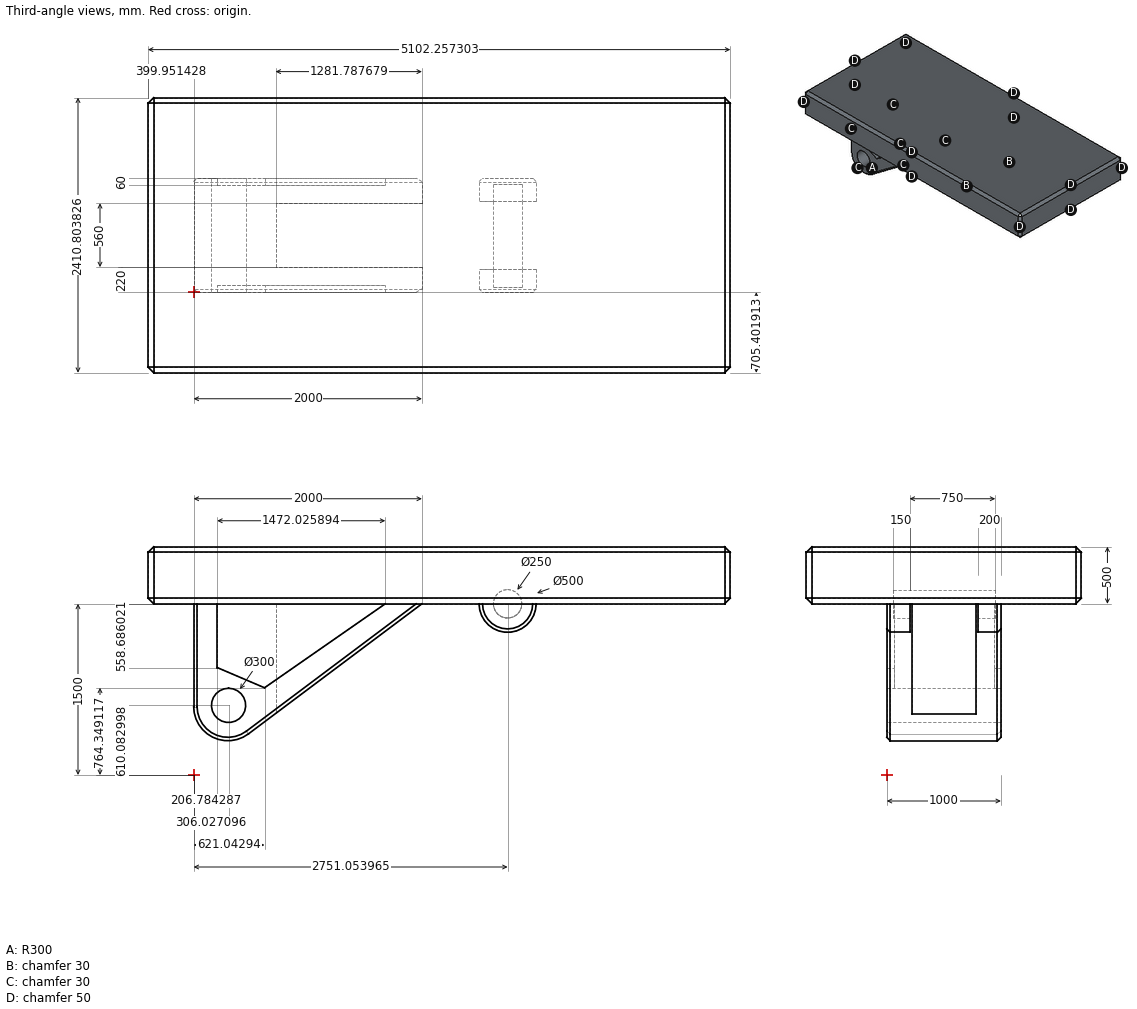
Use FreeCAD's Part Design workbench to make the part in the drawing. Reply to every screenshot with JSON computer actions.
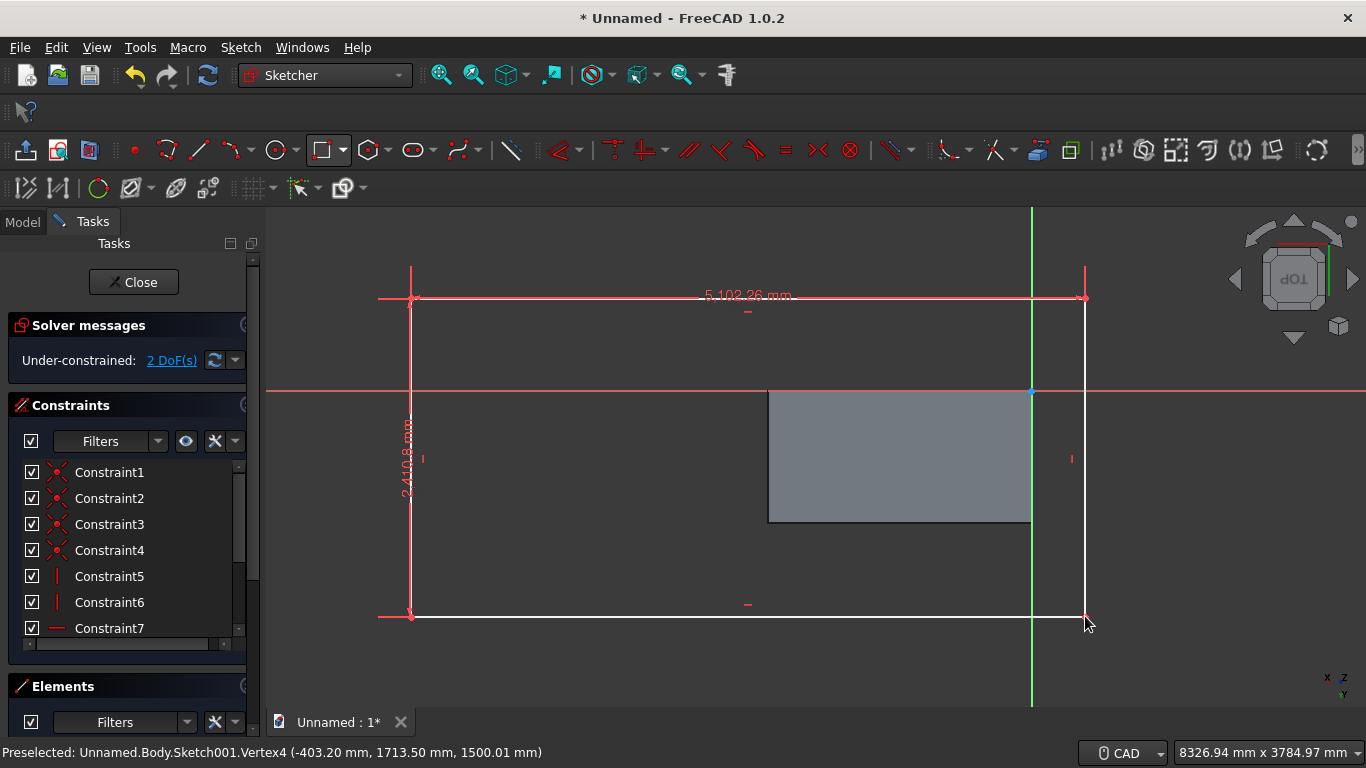
{"action": "key", "text": "d"}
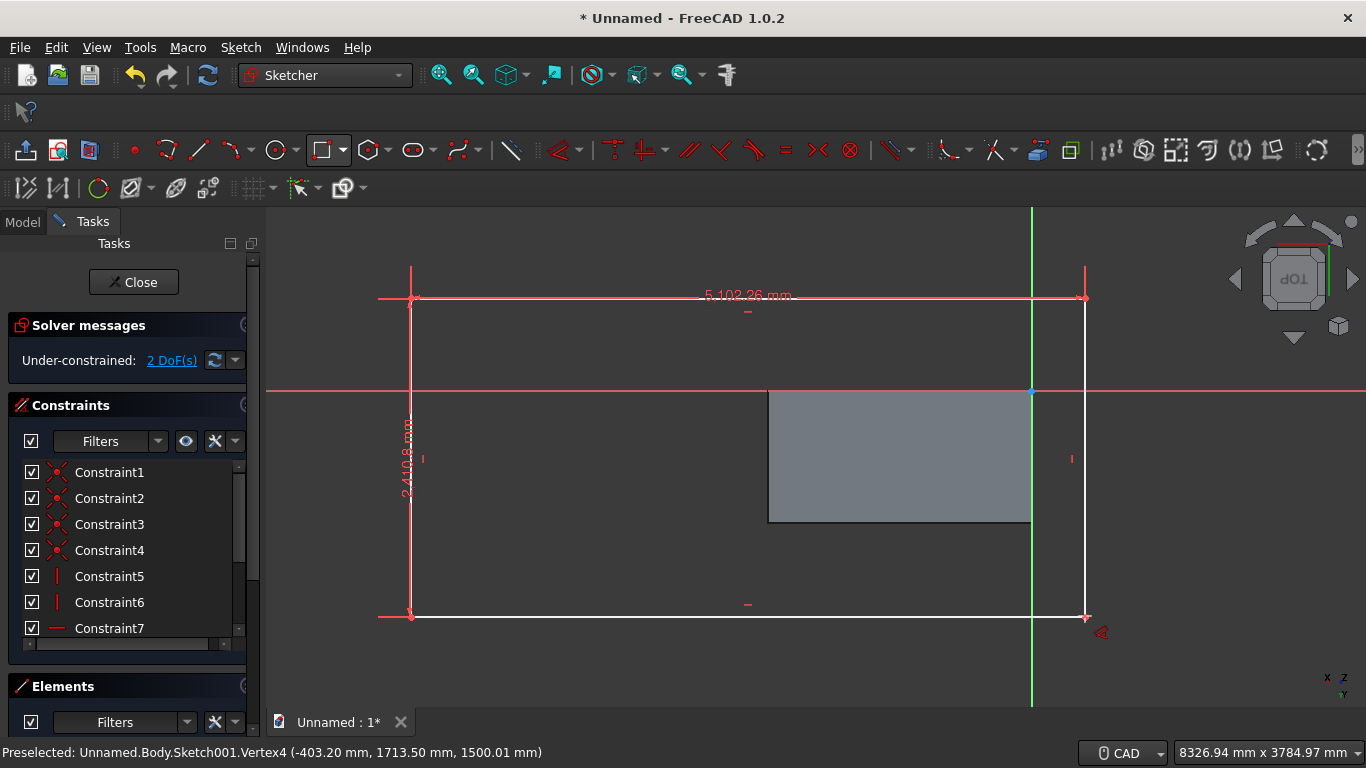
{"action": "left_click", "coordinate": [411, 299]}
{"action": "left_click", "coordinate": [377, 345]}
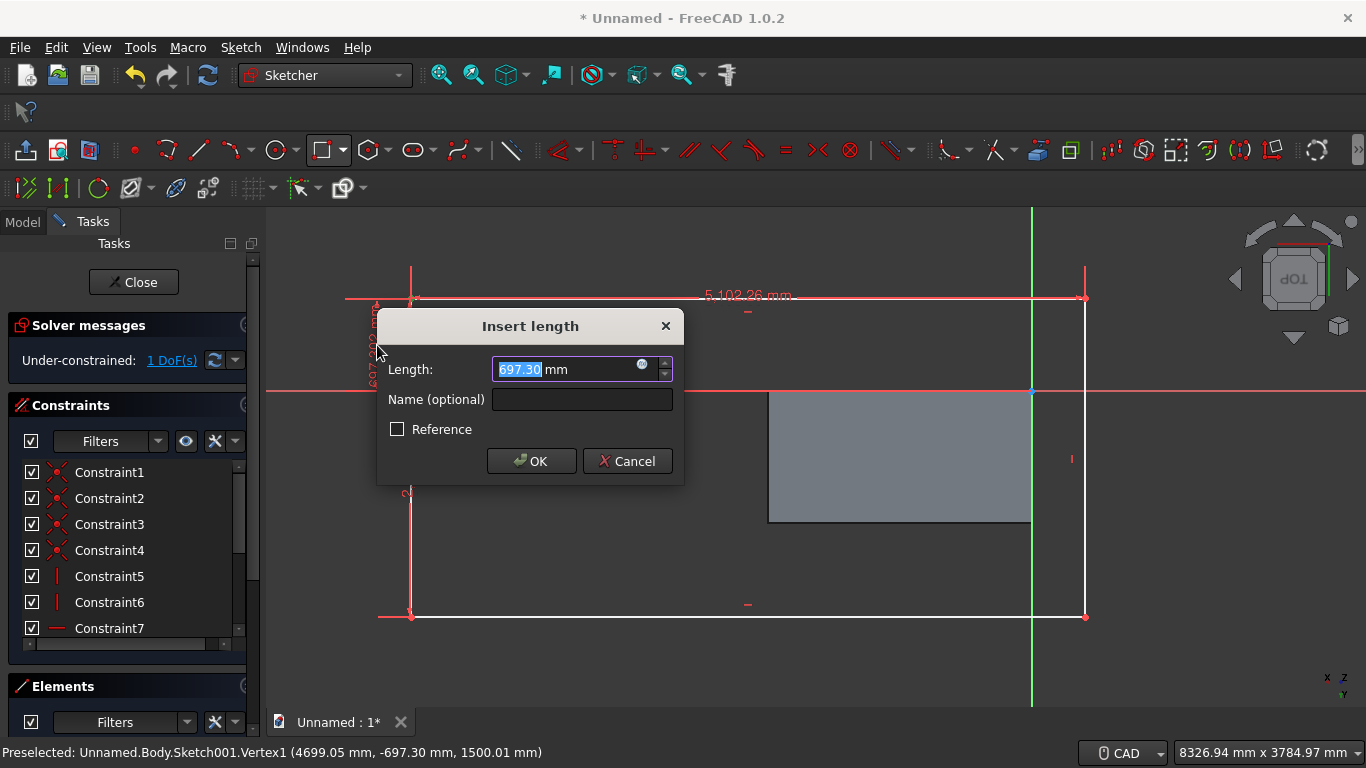
{"action": "type", "text": "705.401913"}
{"action": "key", "text": "Return"}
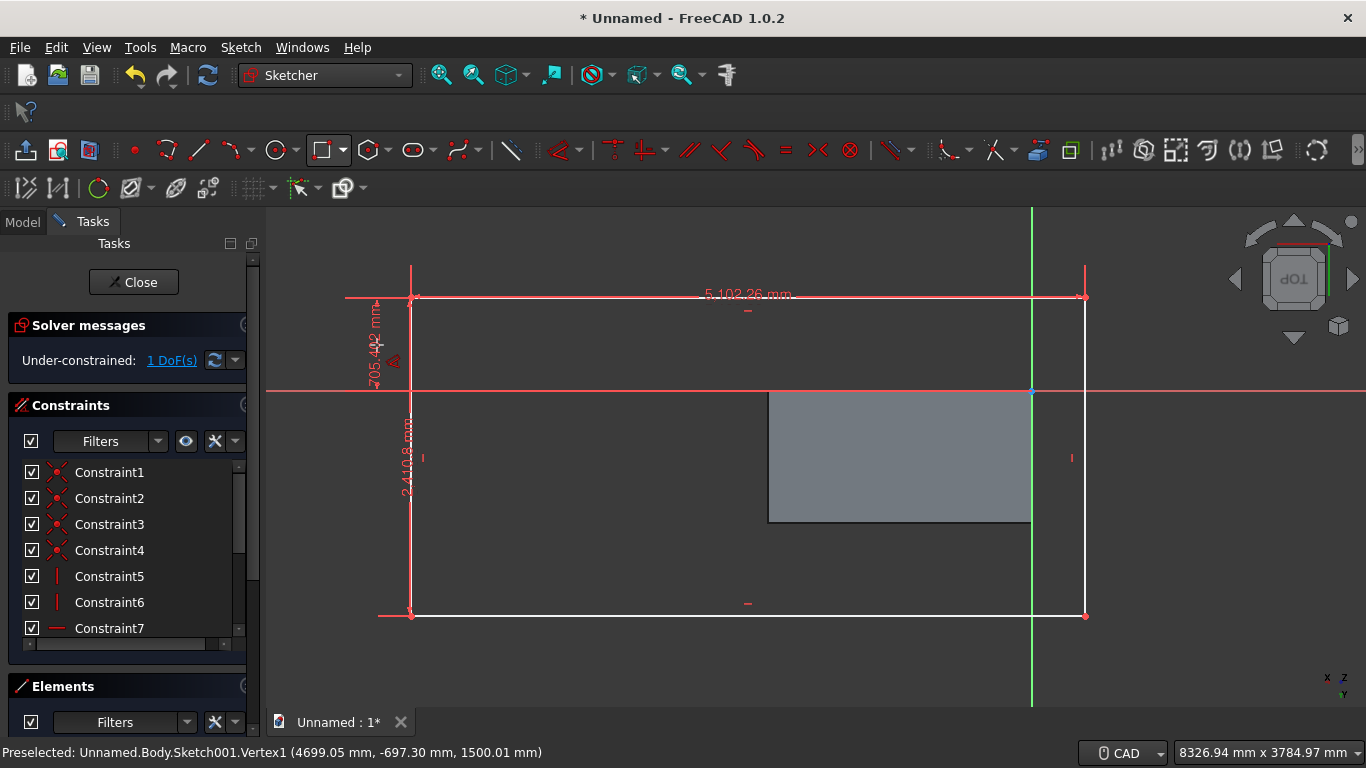
{"action": "left_click", "coordinate": [1085, 616]}
{"action": "left_click", "coordinate": [1058, 650]}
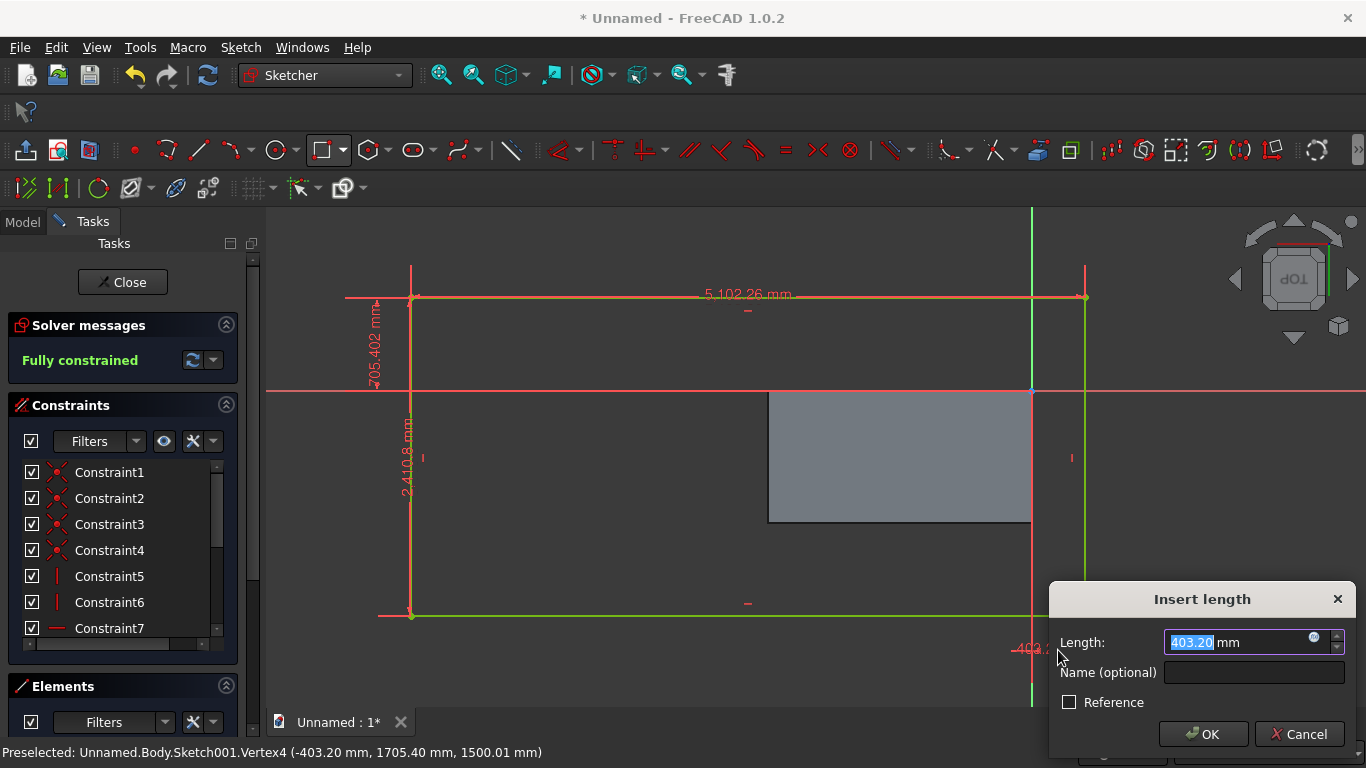
{"action": "type", "text": "399.951428"}
{"action": "key", "text": "Return"}
{"action": "key", "text": "Escape"}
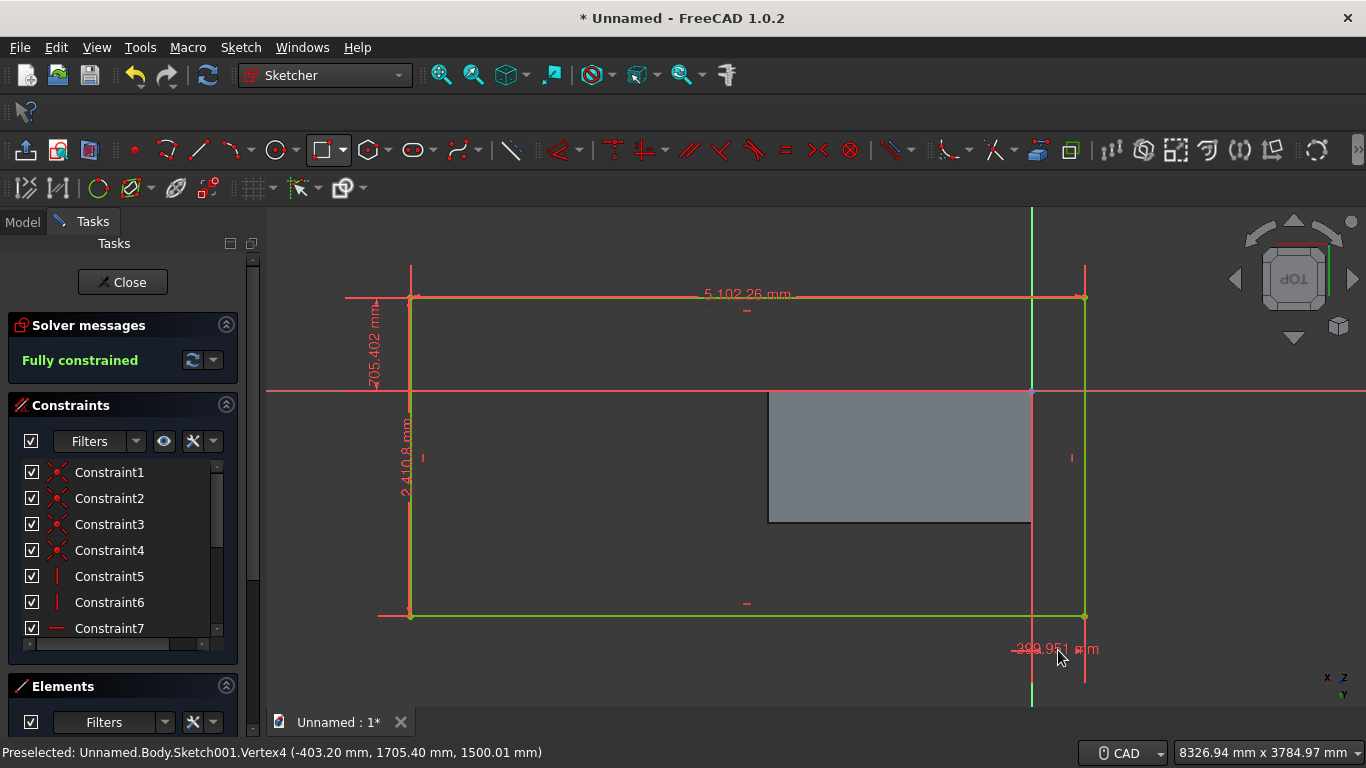
{"action": "left_click", "coordinate": [123, 282]}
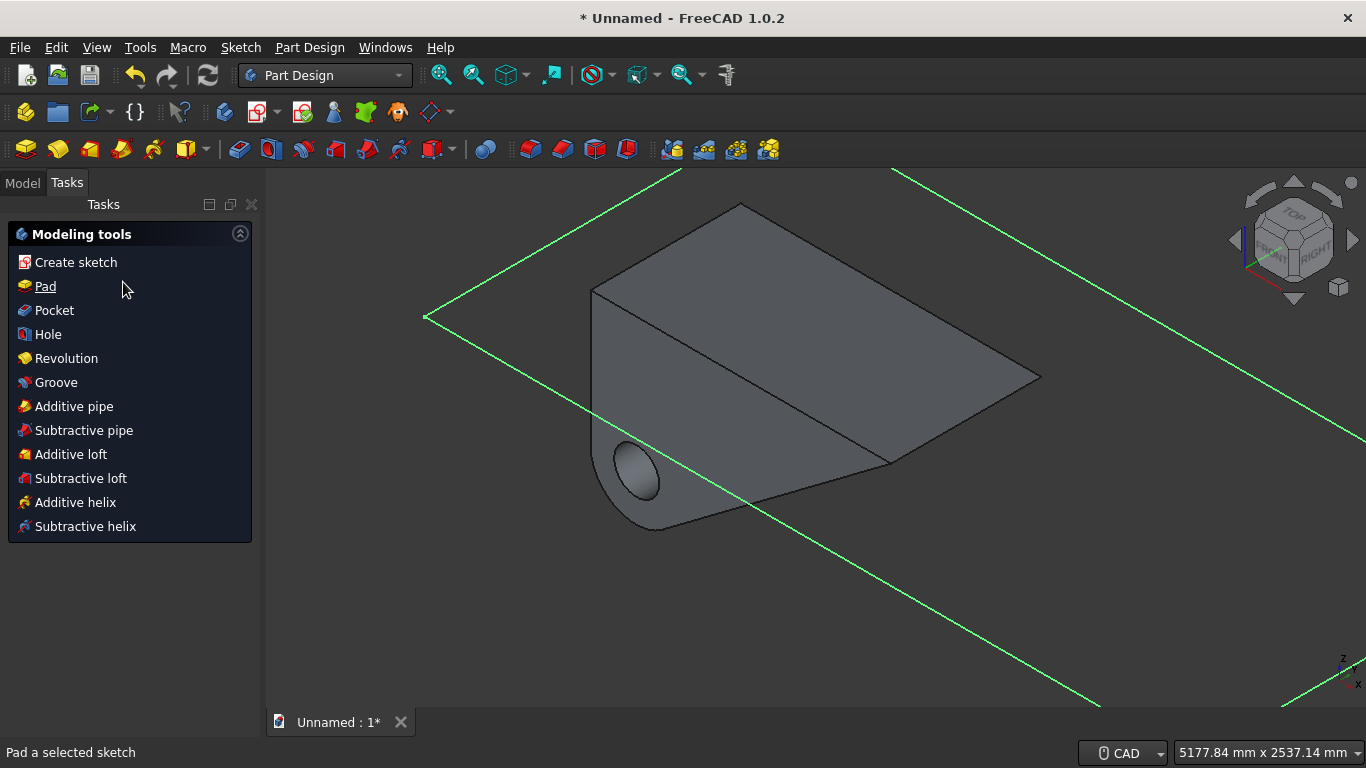
{"action": "left_click", "coordinate": [26, 150]}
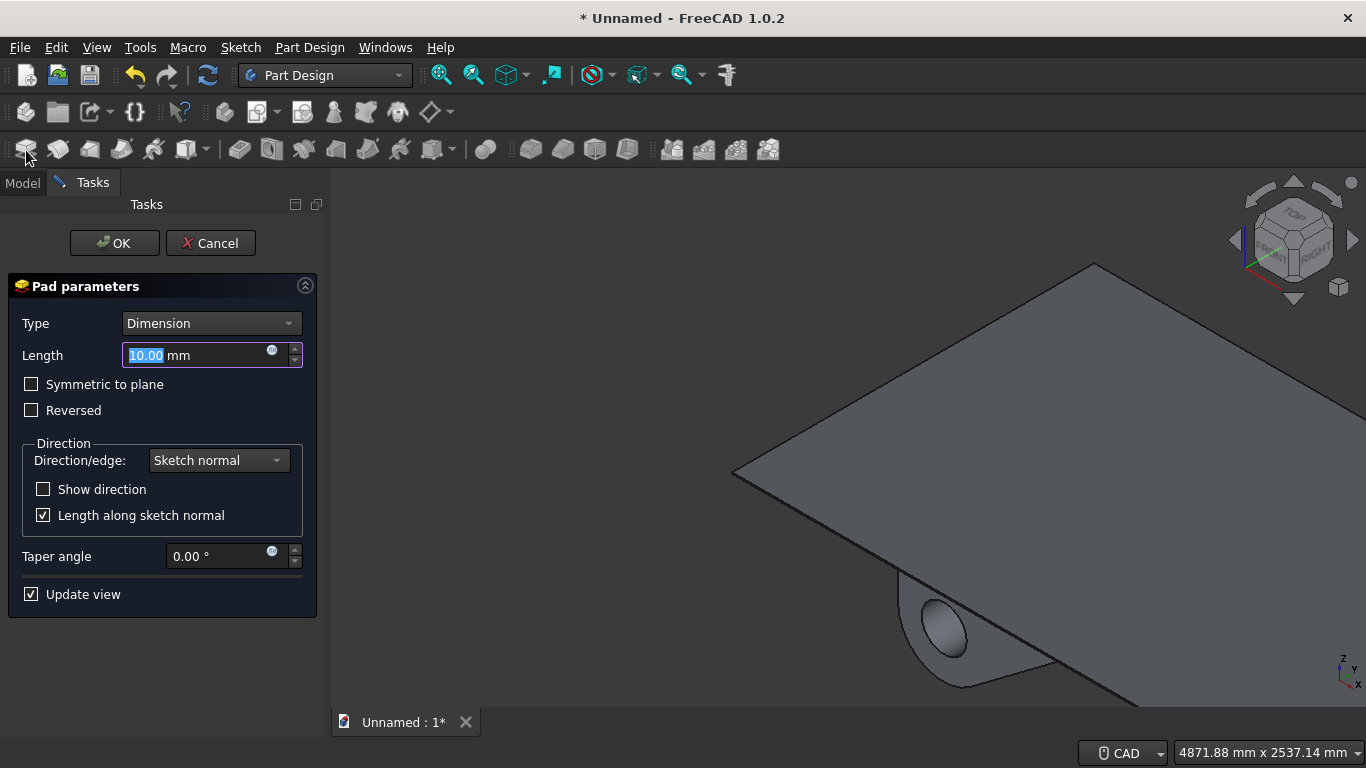
{"action": "type", "text": "500"}
{"action": "key", "text": "Tab"}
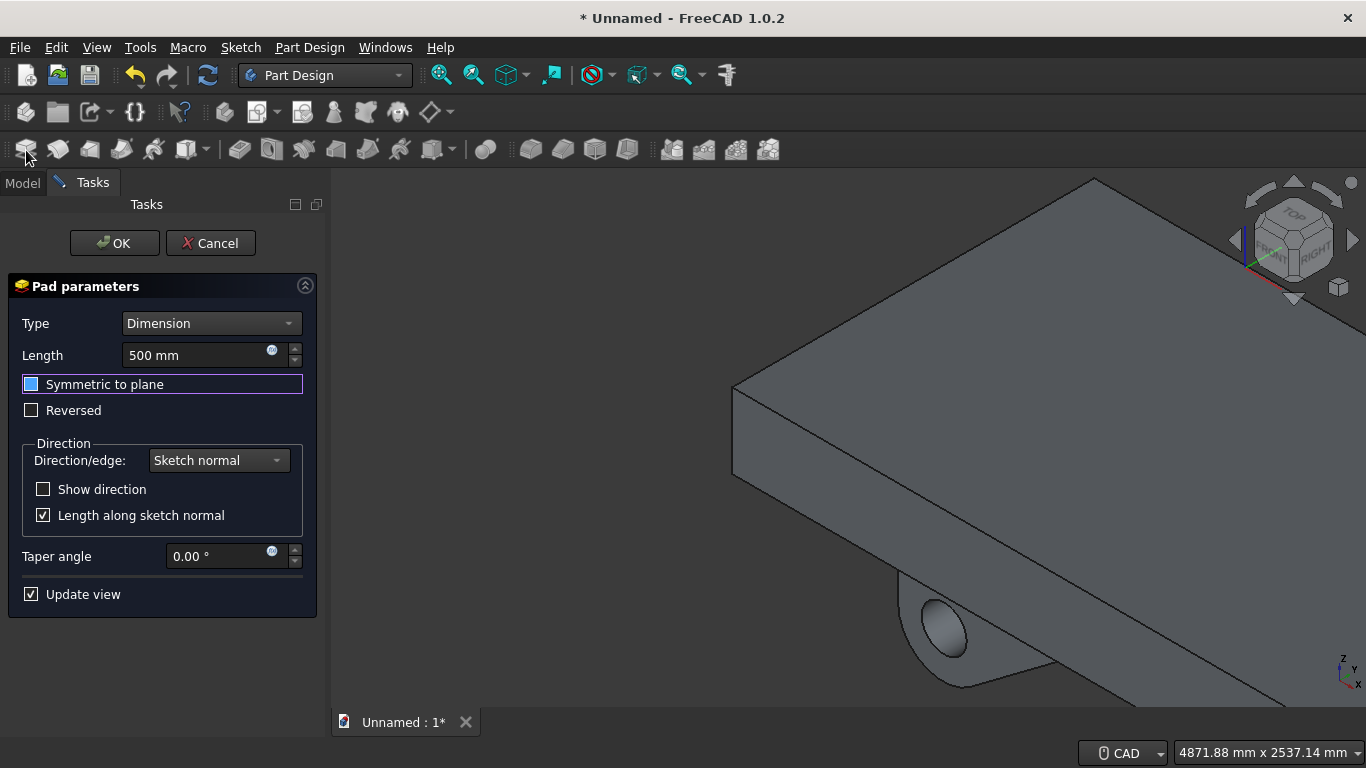
{"action": "left_click", "coordinate": [115, 243]}